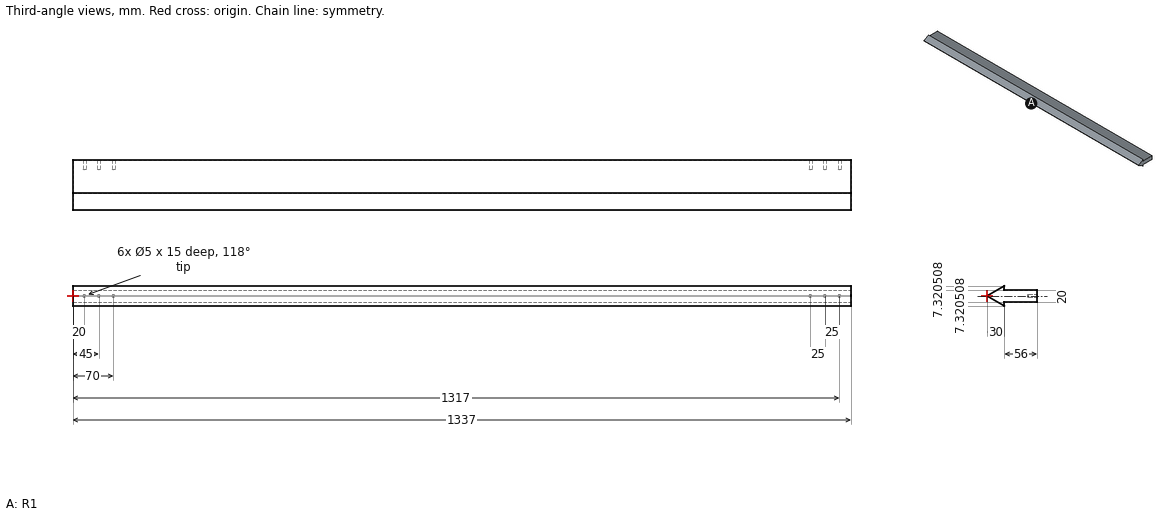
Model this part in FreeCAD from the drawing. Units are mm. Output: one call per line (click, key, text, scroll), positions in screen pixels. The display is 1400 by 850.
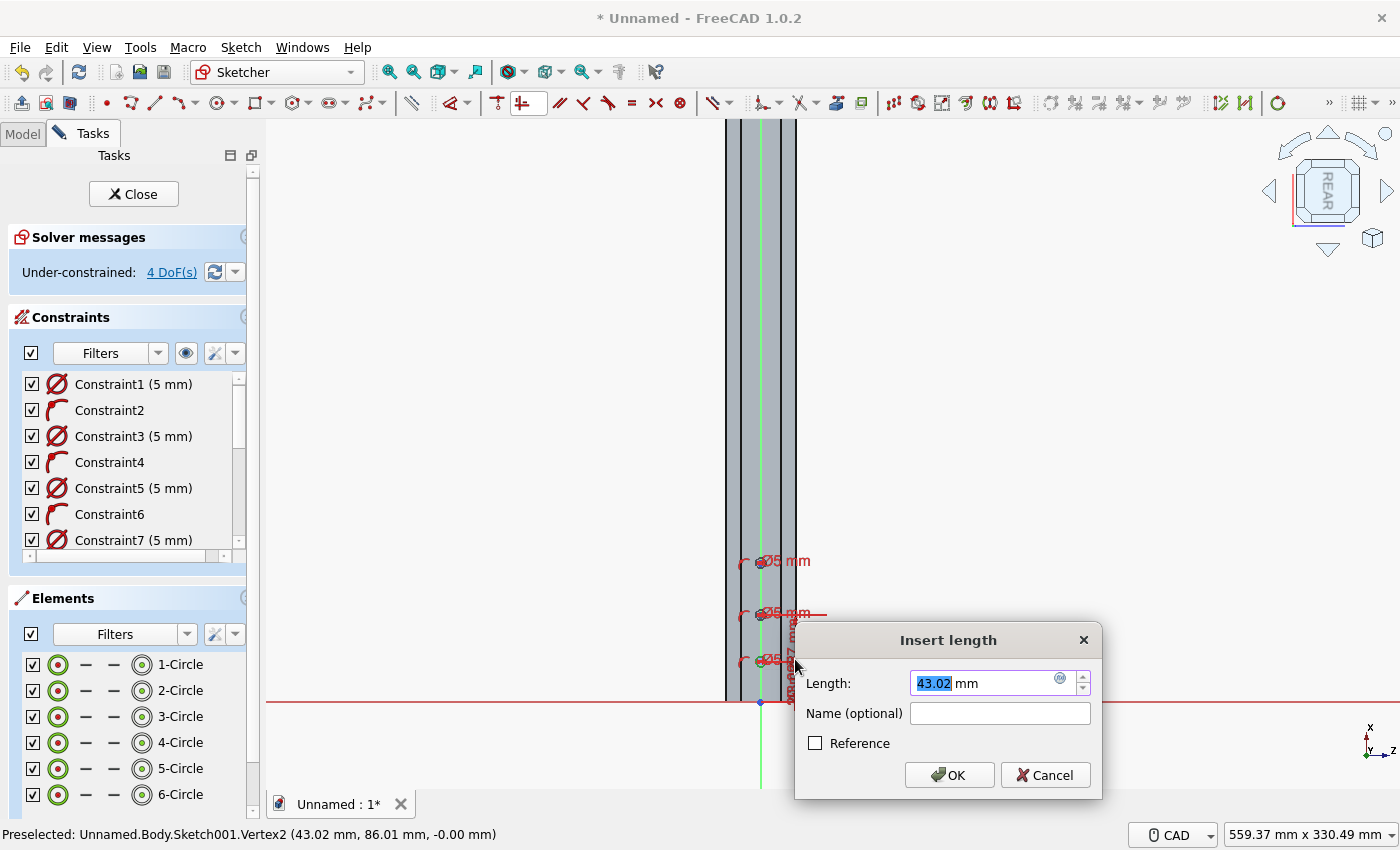
text(45)
key(Return)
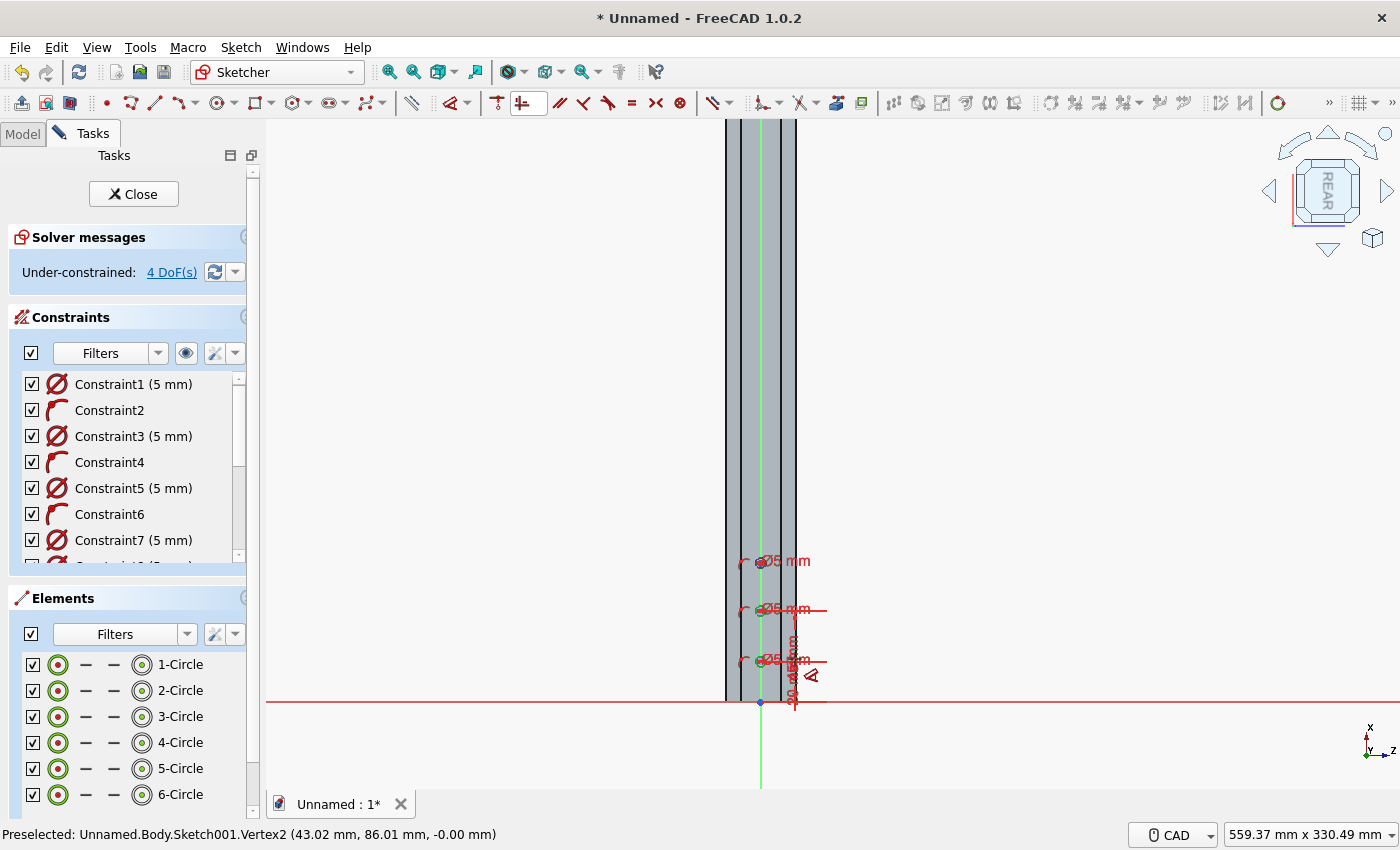
scroll(765, 670, down, 9)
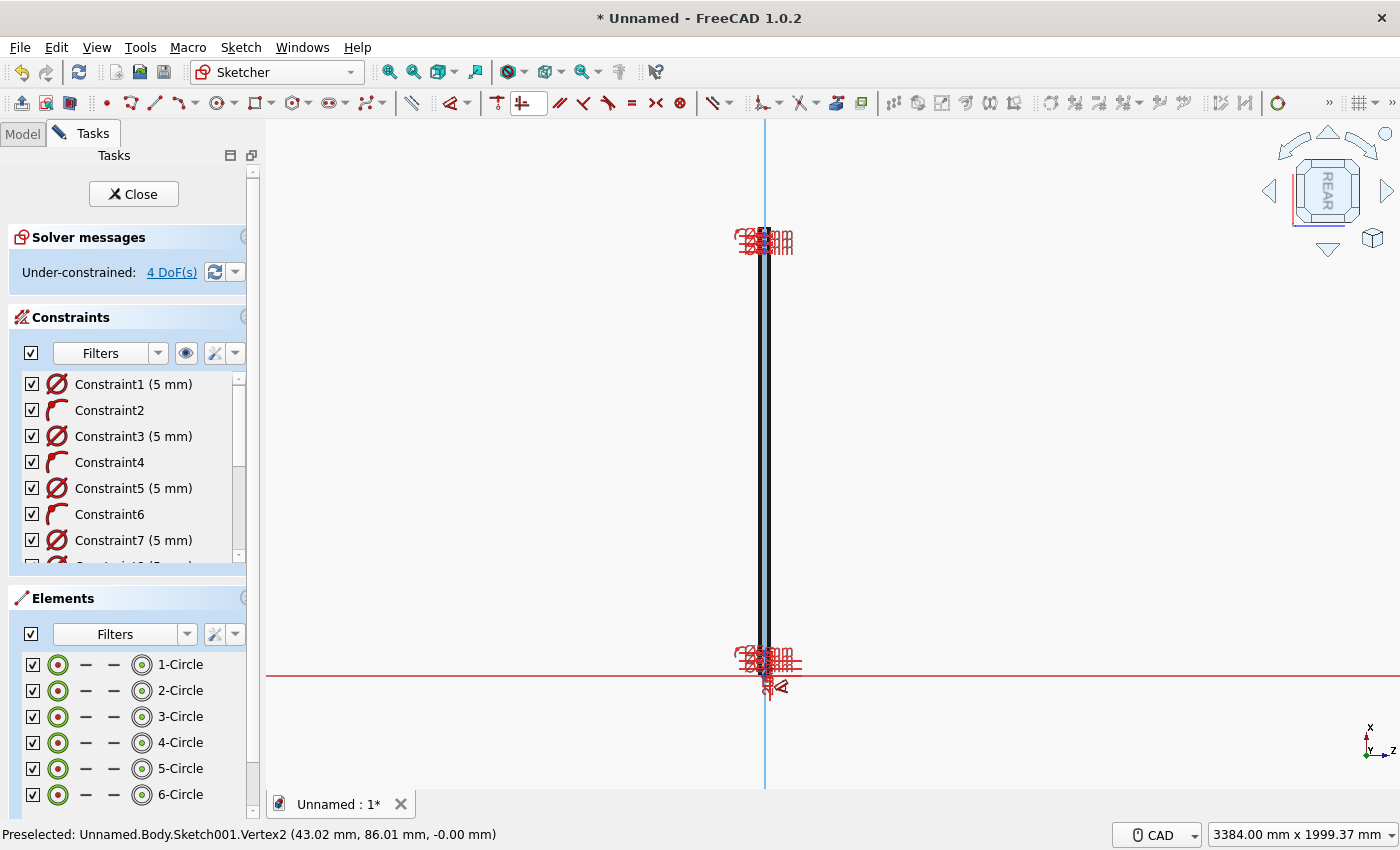
scroll(765, 653, up, 3)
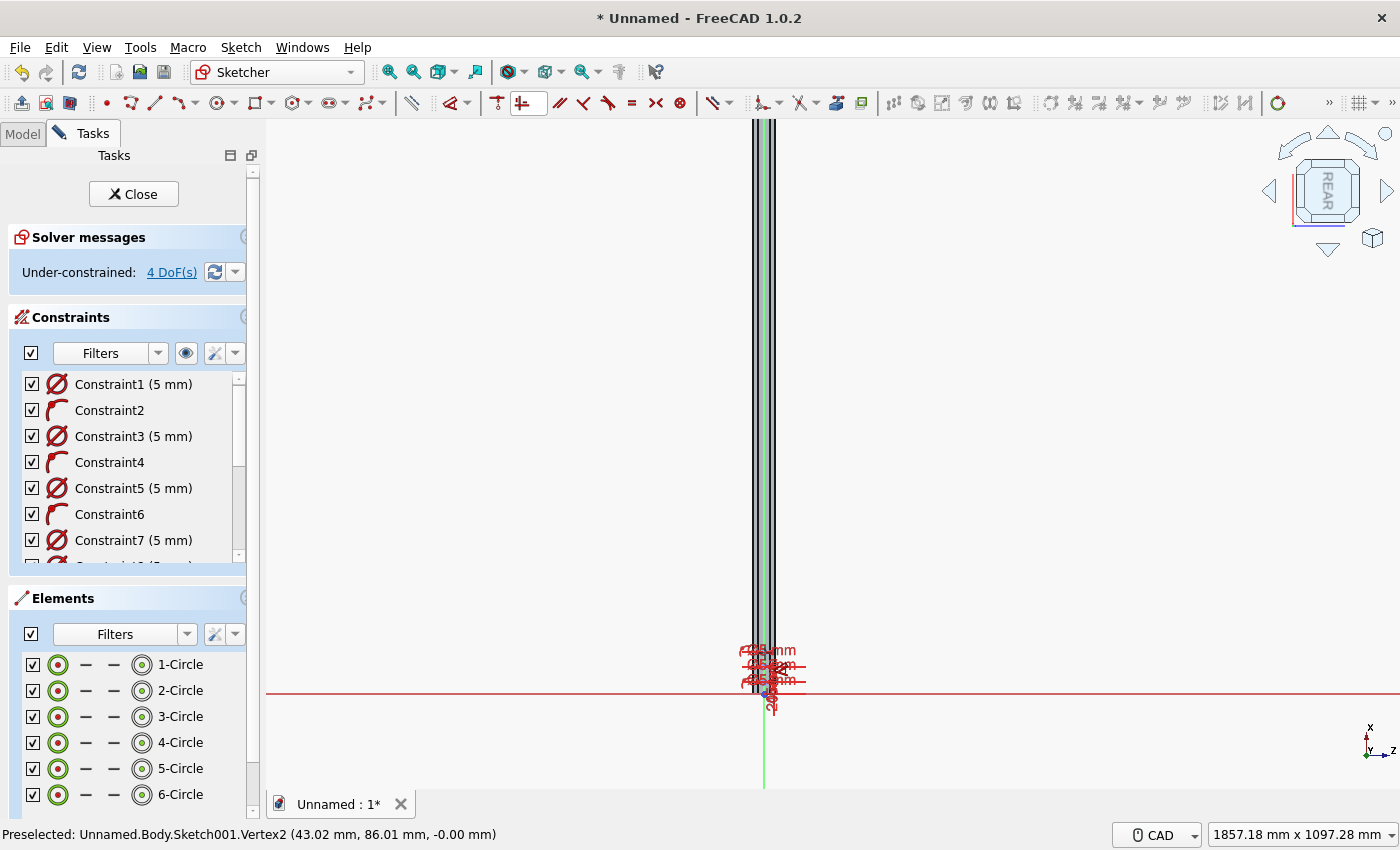
click(764, 652)
click(798, 659)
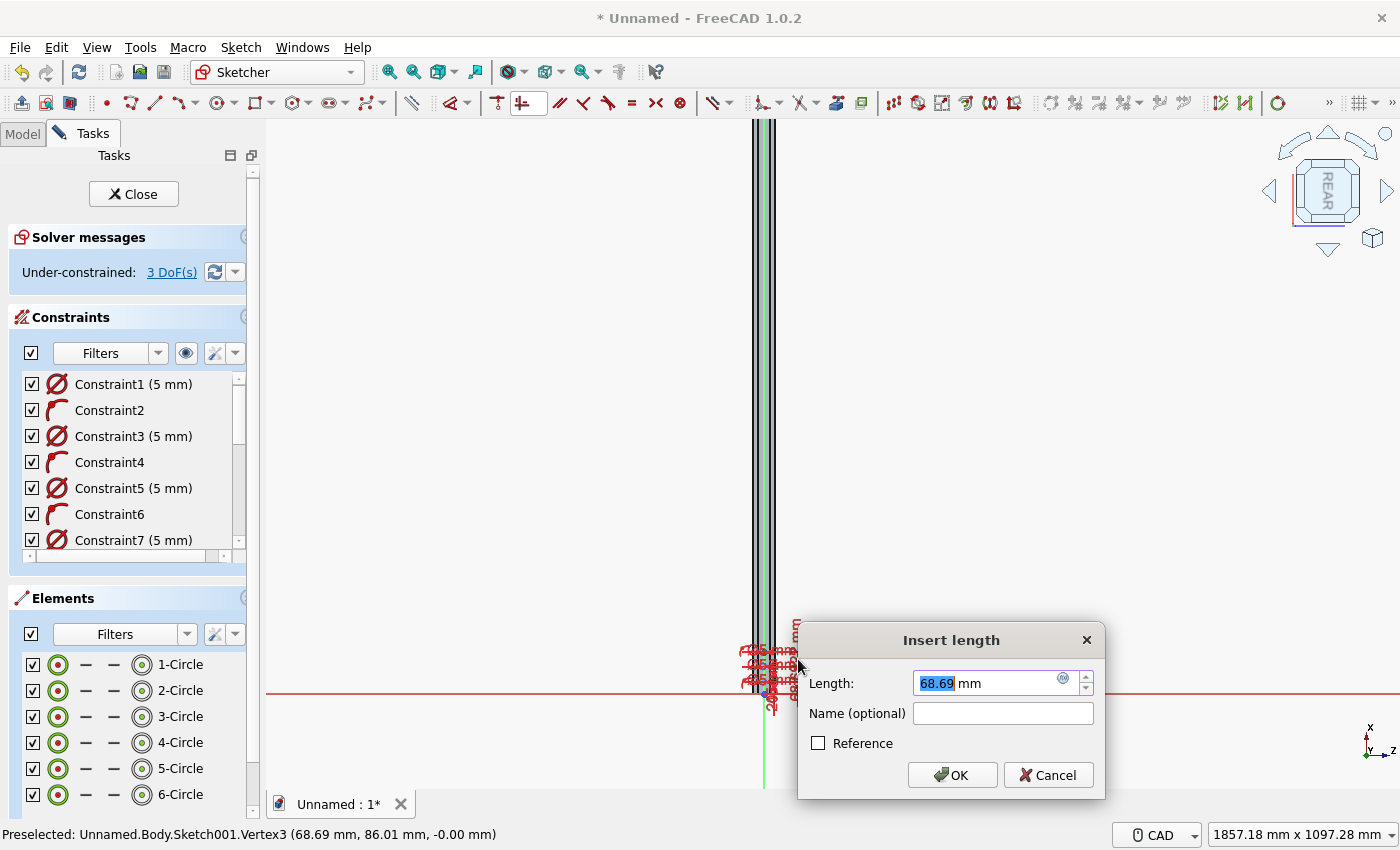
text(70)
key(Return)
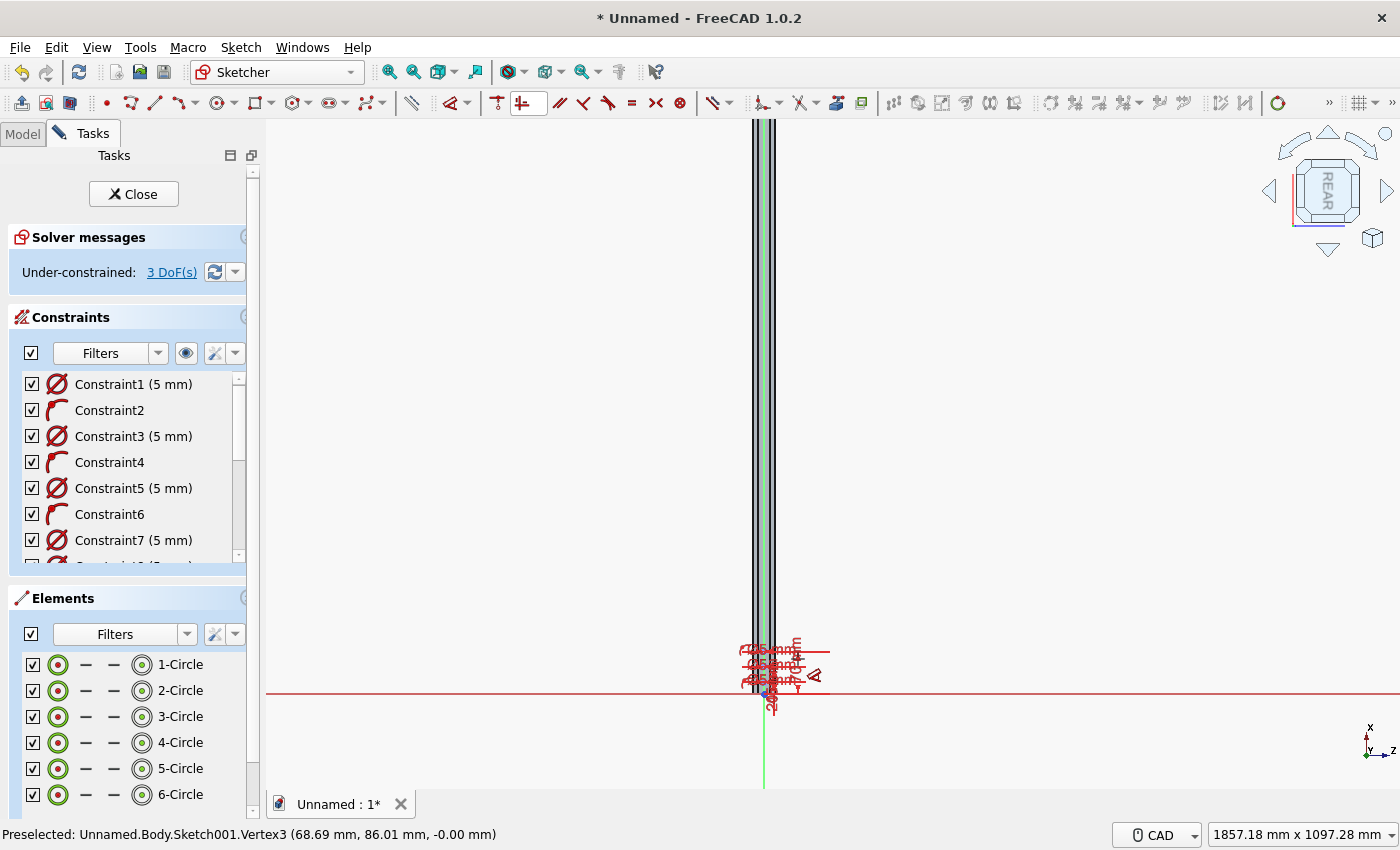
scroll(765, 652, down, 3)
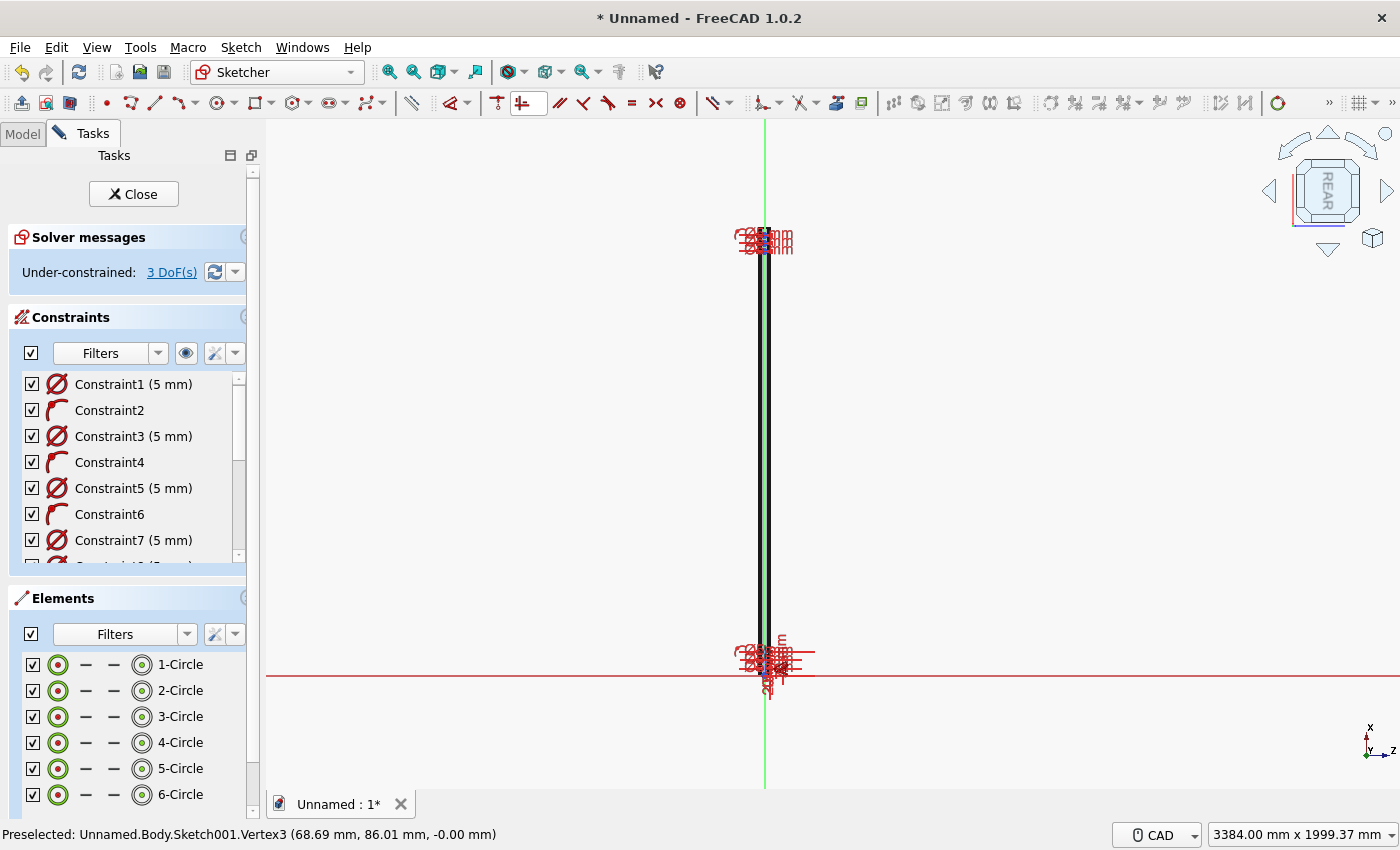
scroll(765, 235, up, 8)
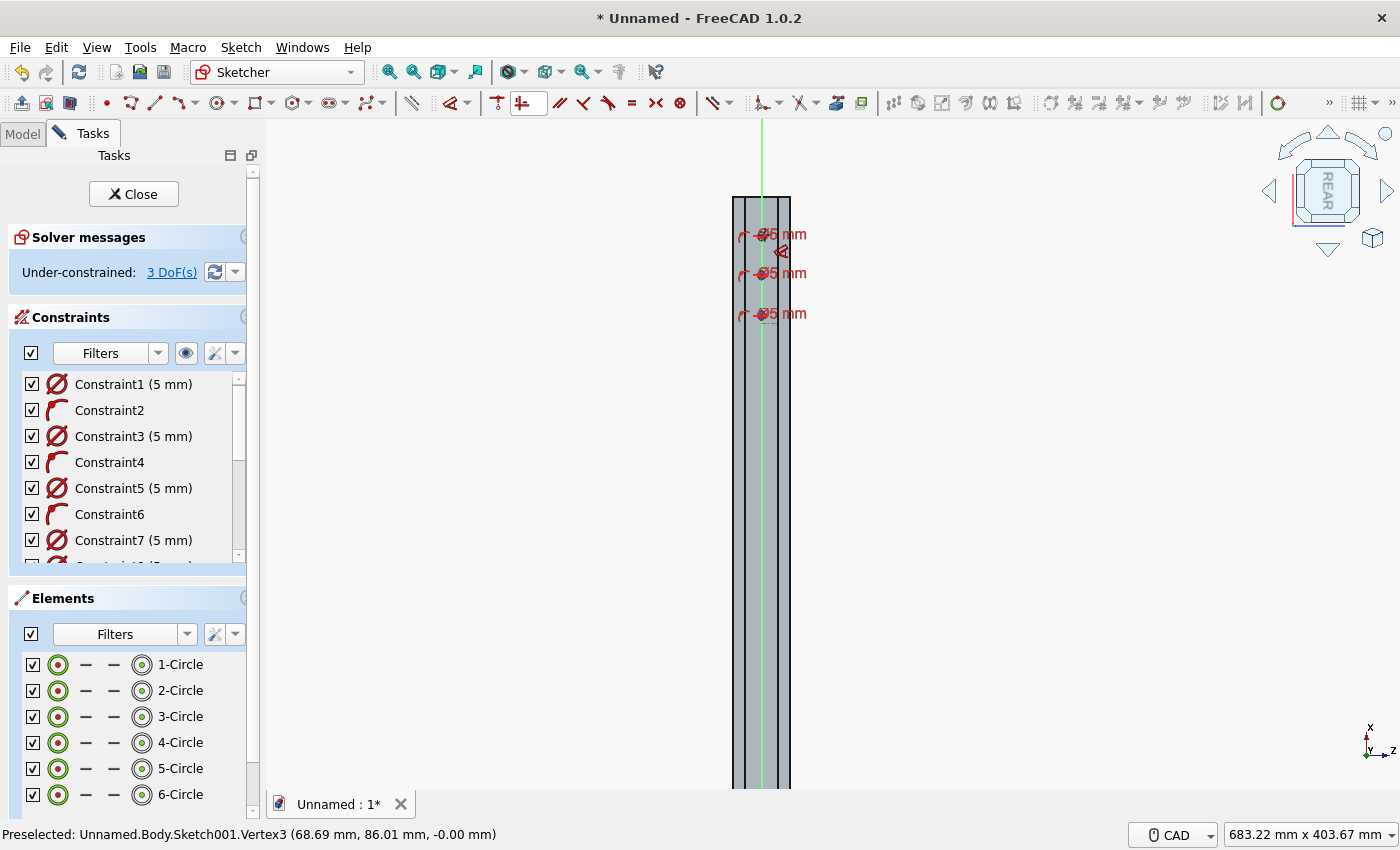
click(762, 236)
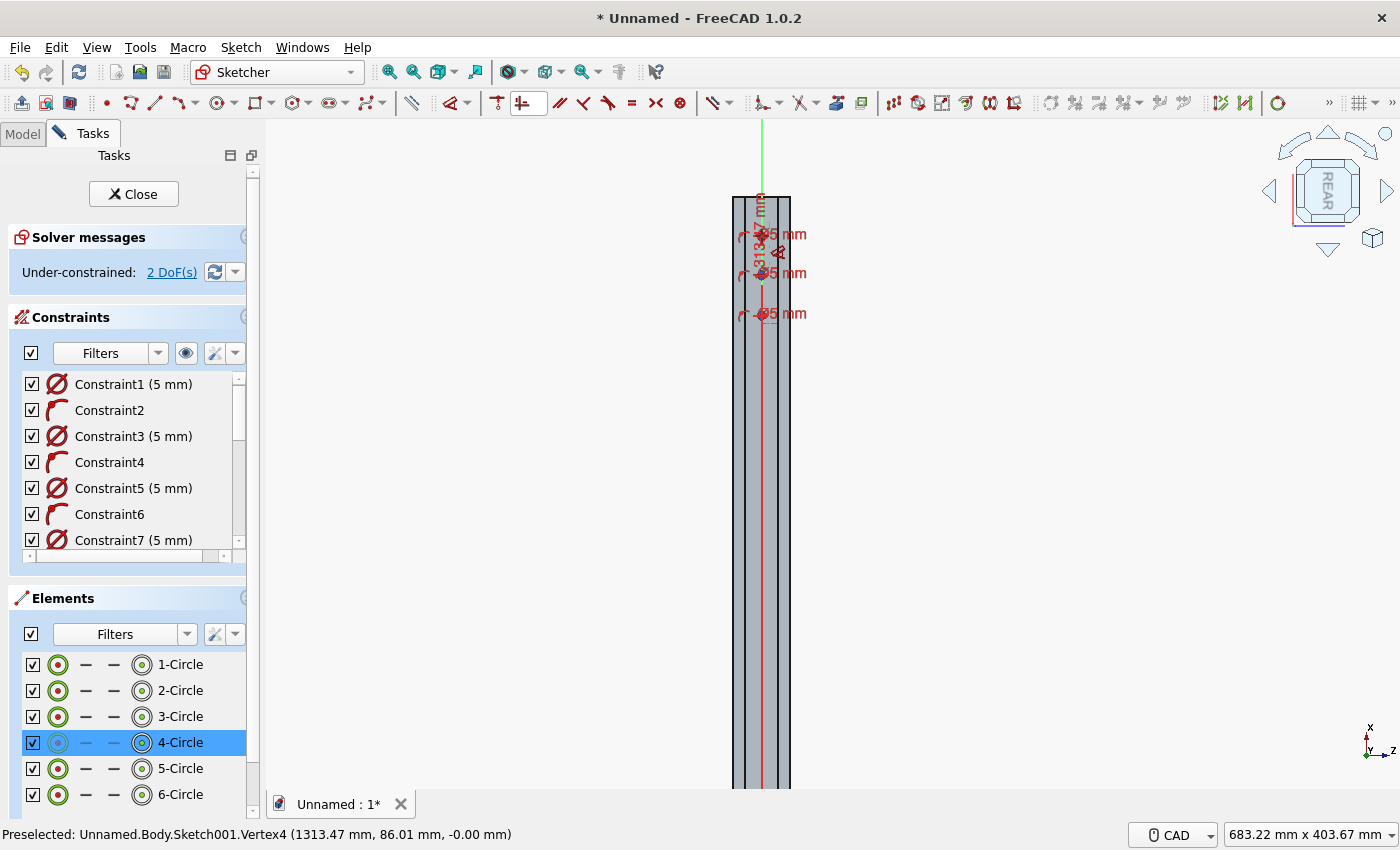
click(762, 275)
click(796, 256)